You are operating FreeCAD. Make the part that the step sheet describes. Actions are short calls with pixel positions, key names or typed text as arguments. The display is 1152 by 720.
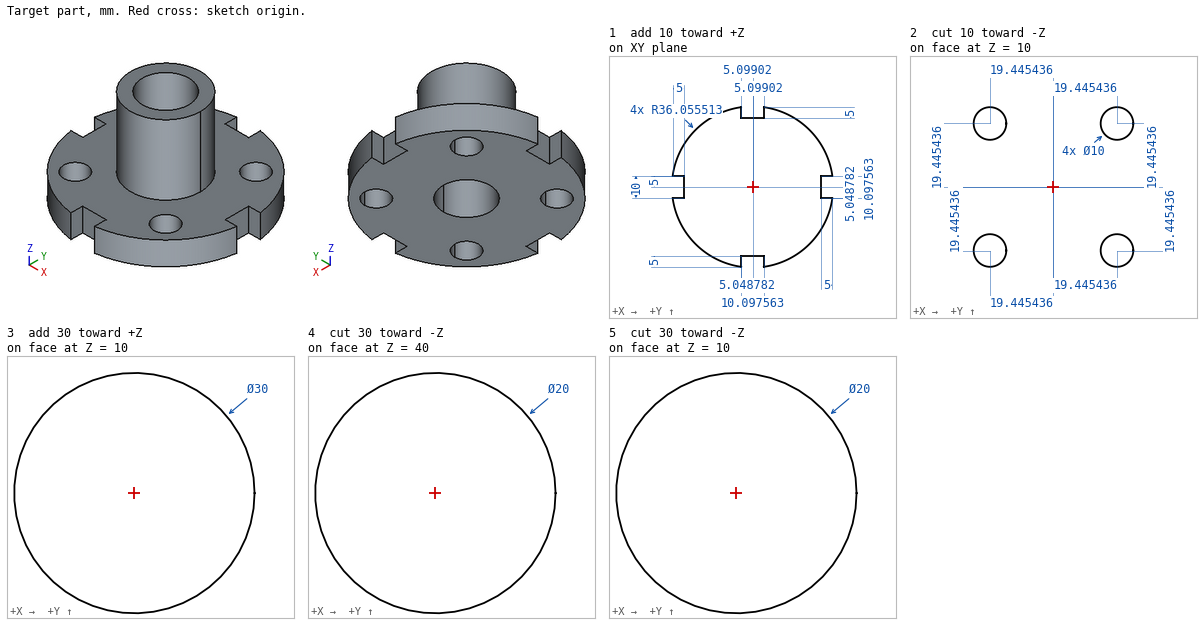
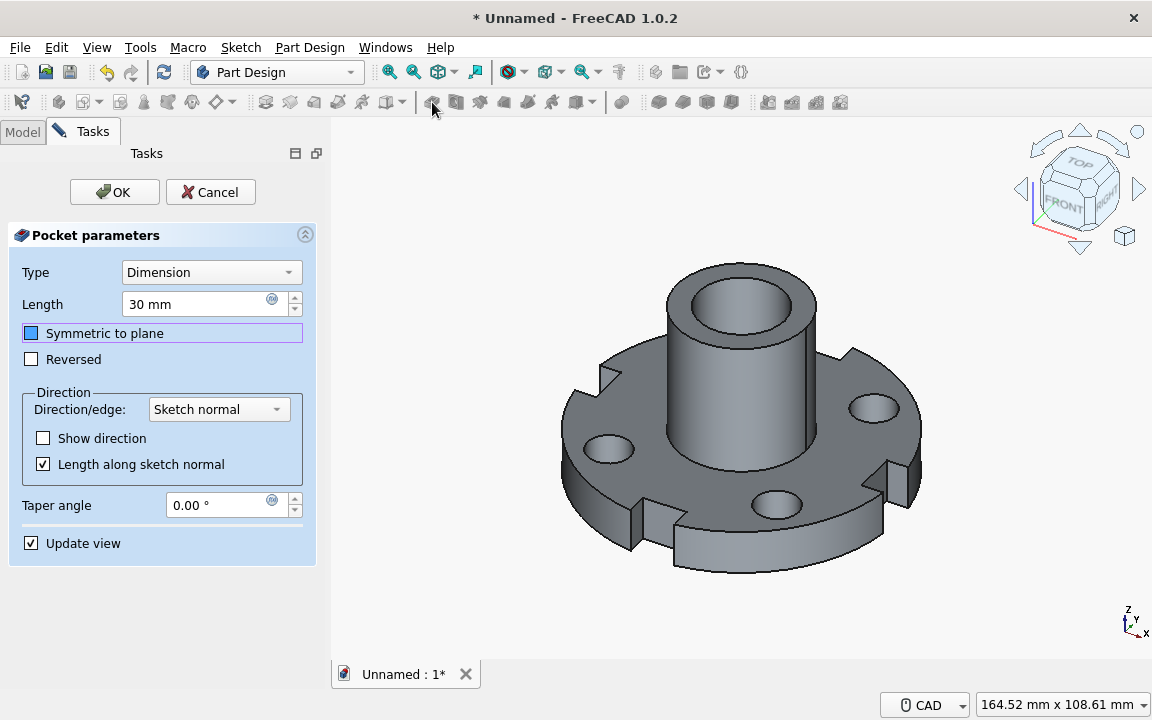
click(115, 192)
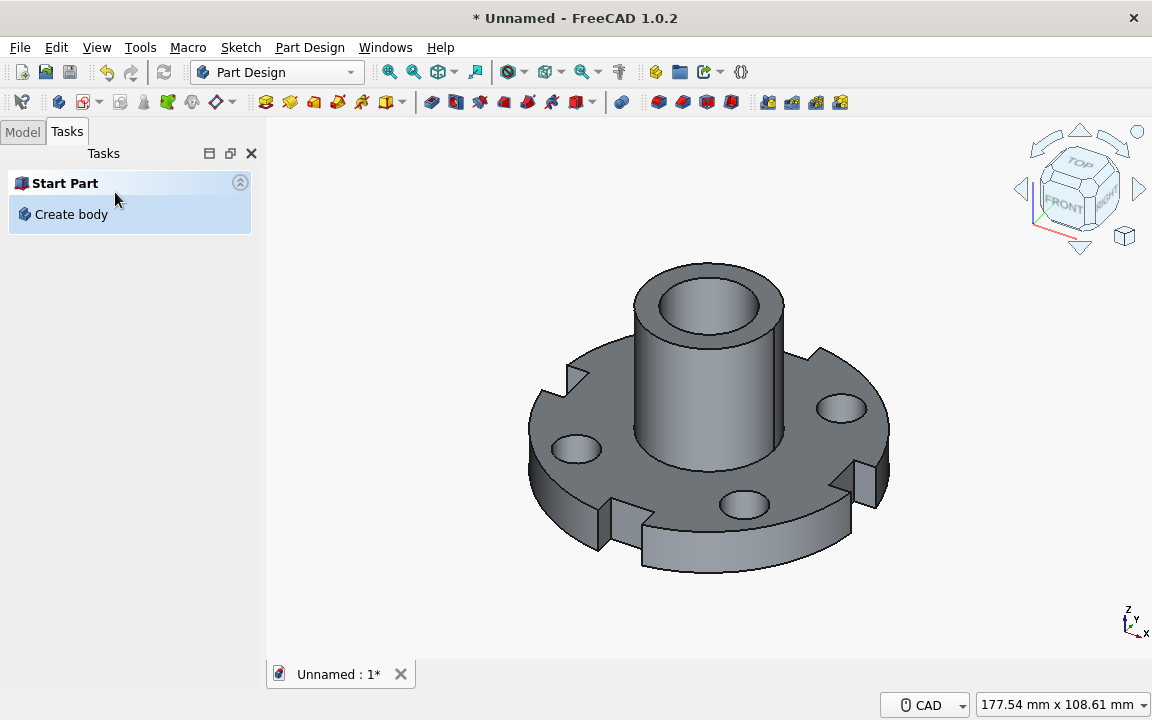
click(621, 399)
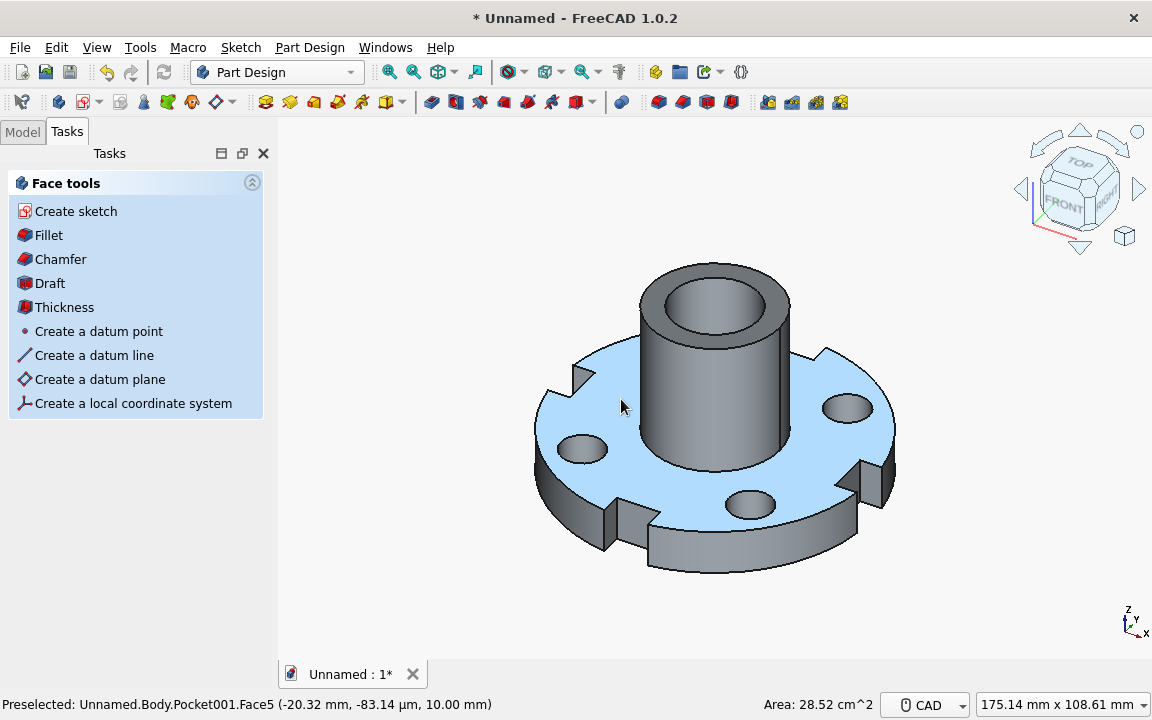
click(84, 102)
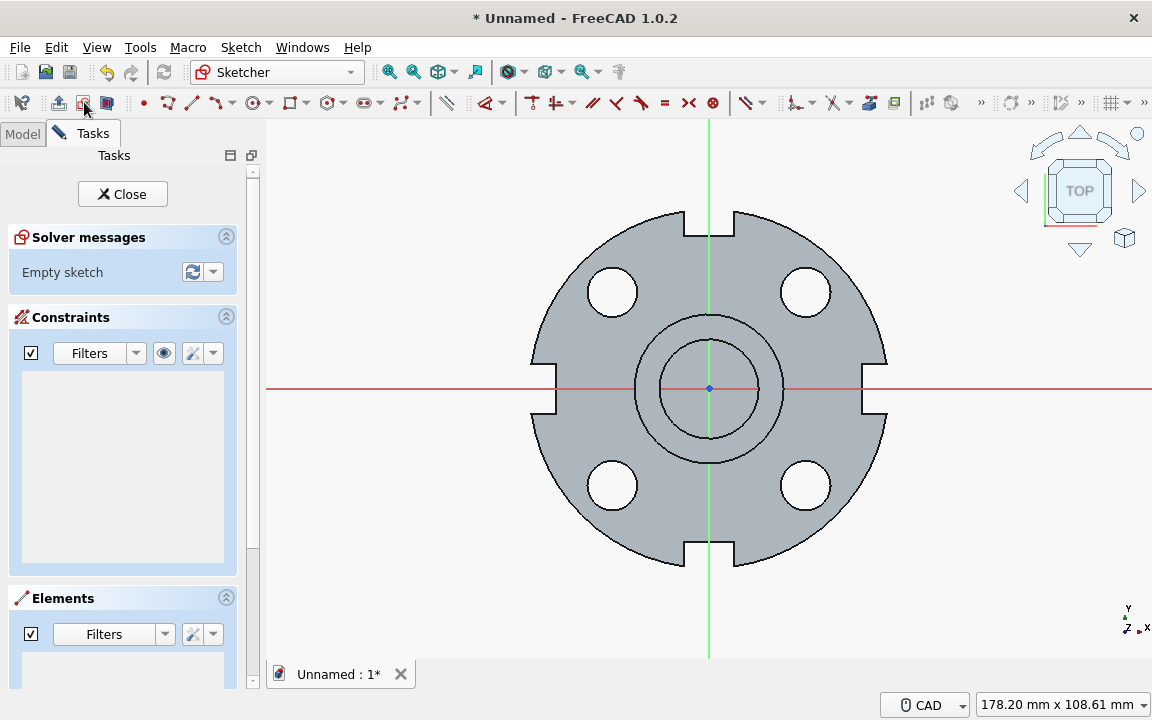
scroll(739, 389, up, 6)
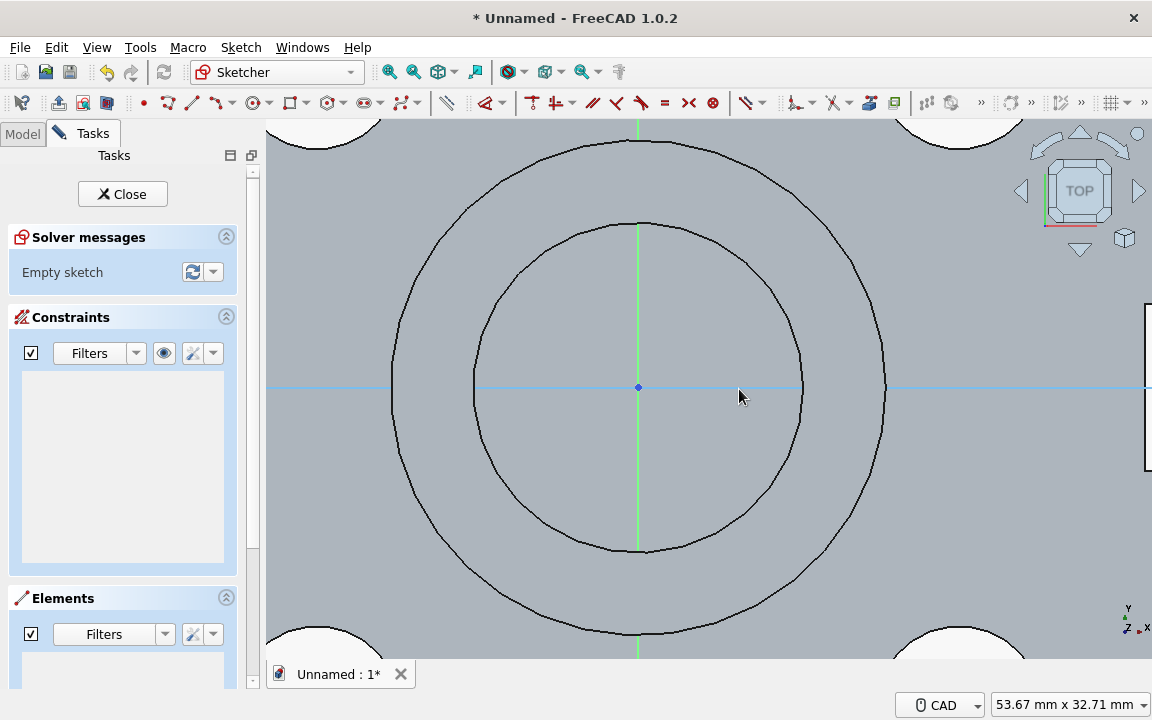
click(254, 104)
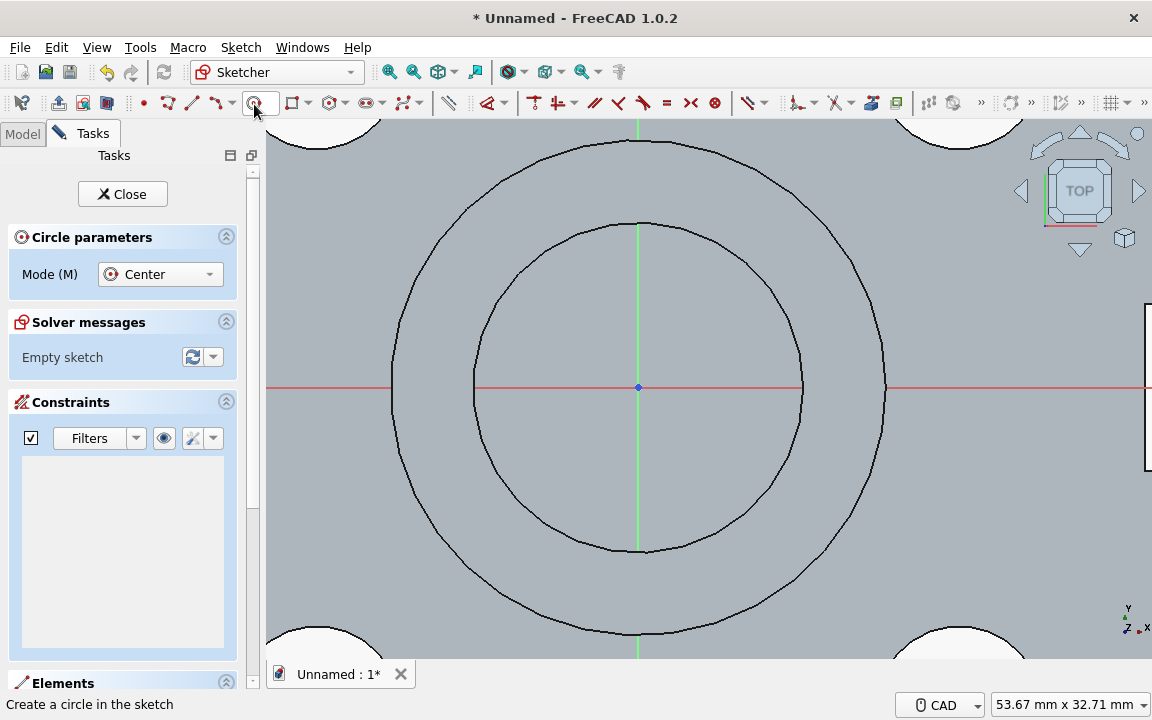
click(638, 388)
move(755, 271)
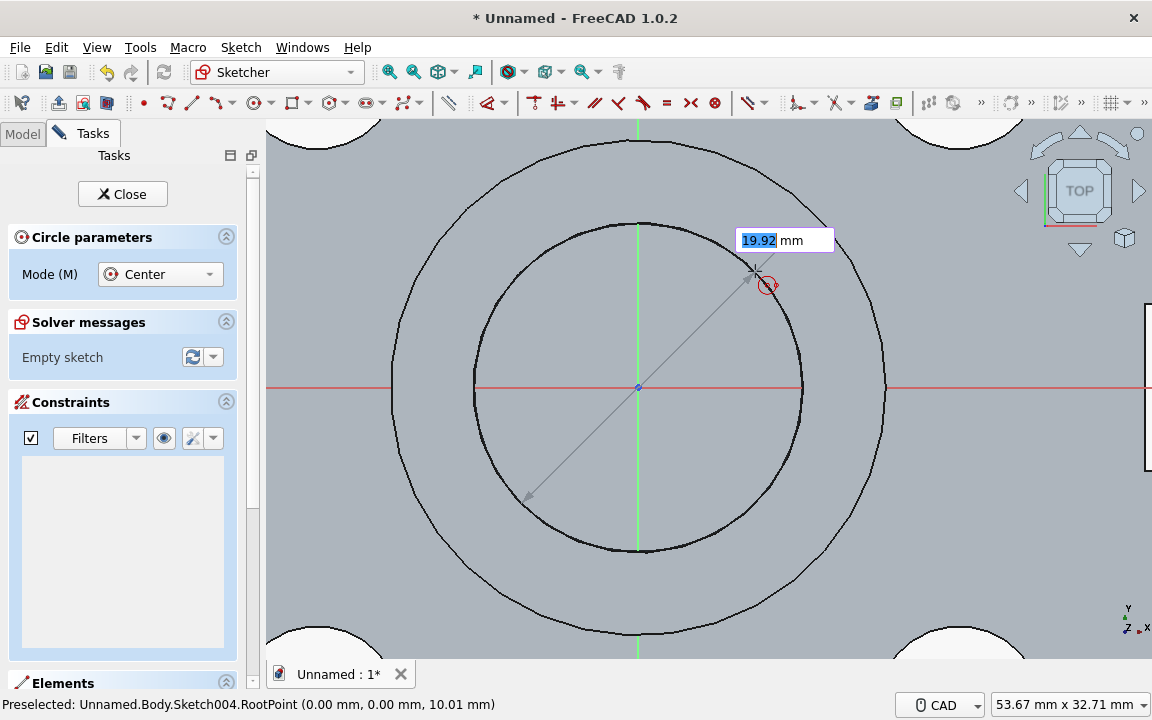
text(20)
key(Return)
key(Escape)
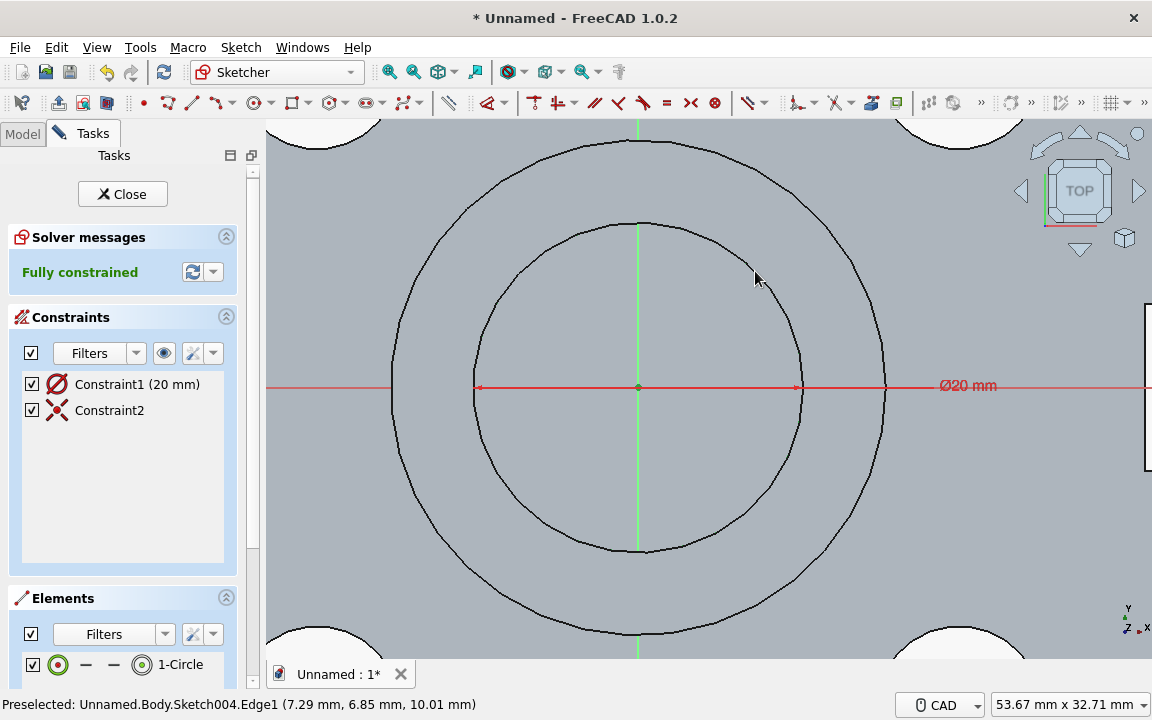
click(123, 194)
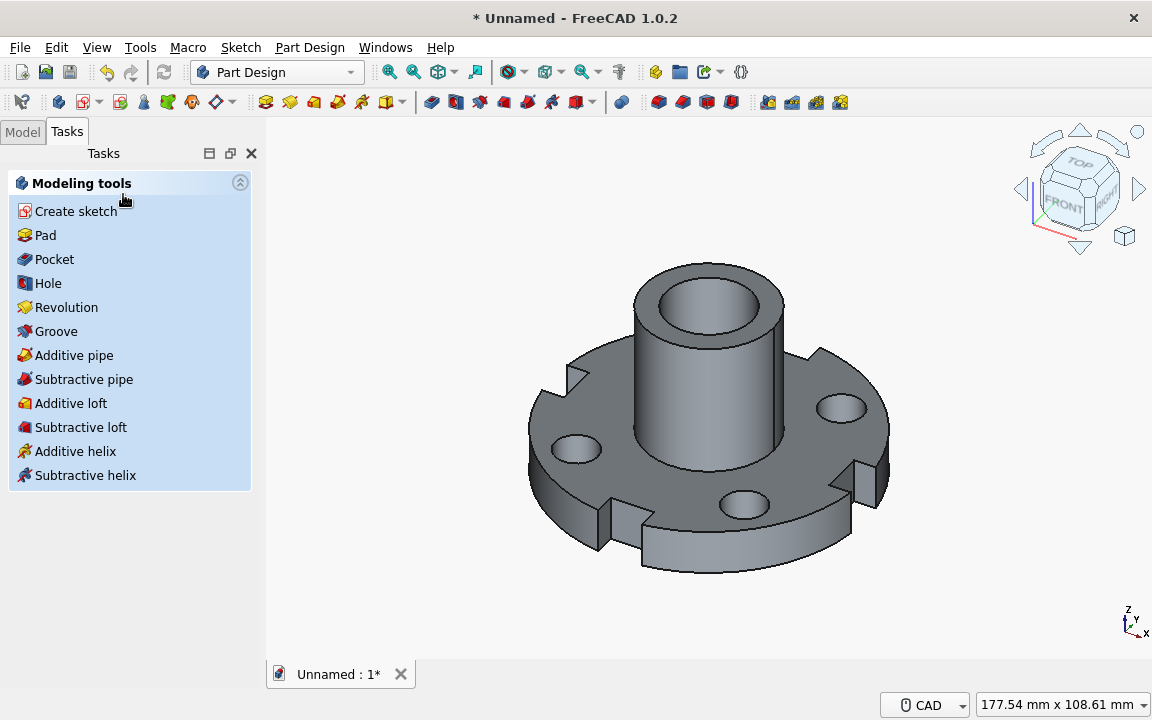
click(432, 102)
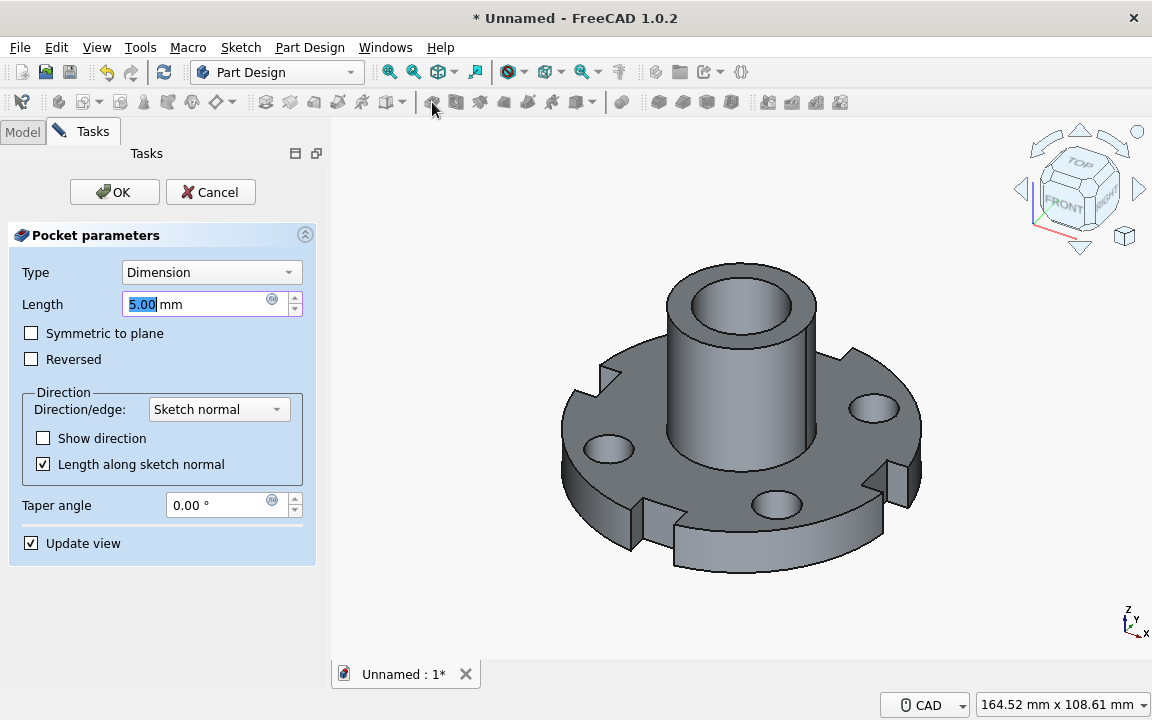
text(30)
key(Tab)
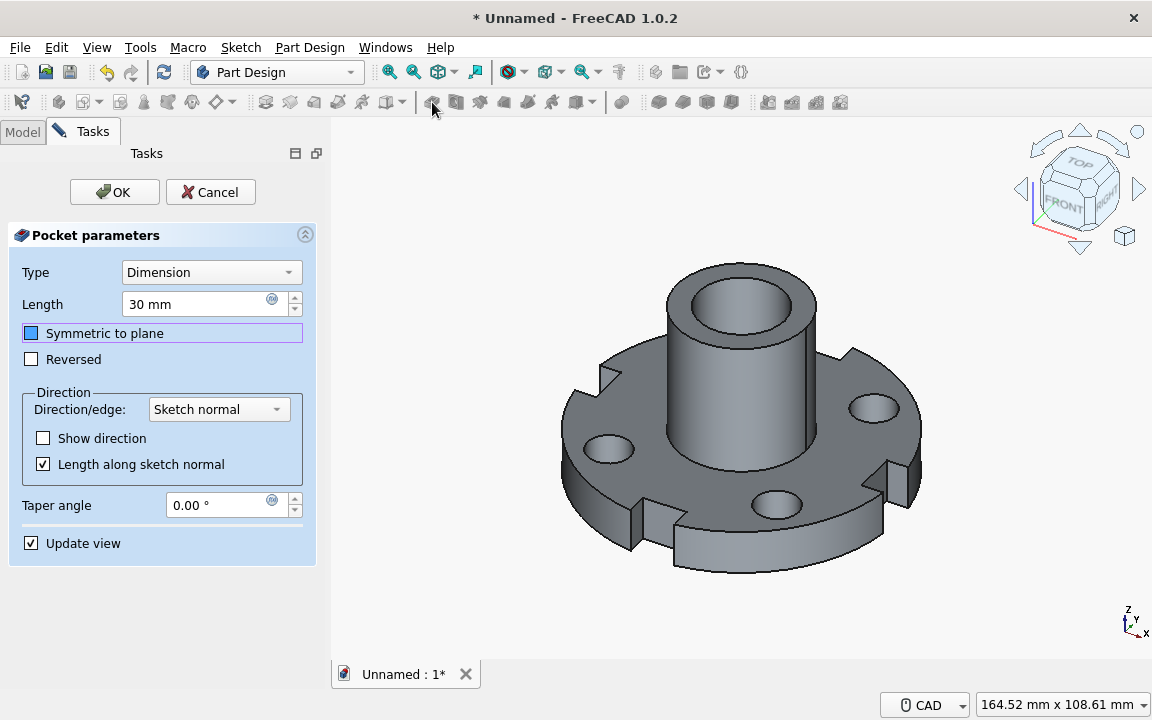
click(115, 192)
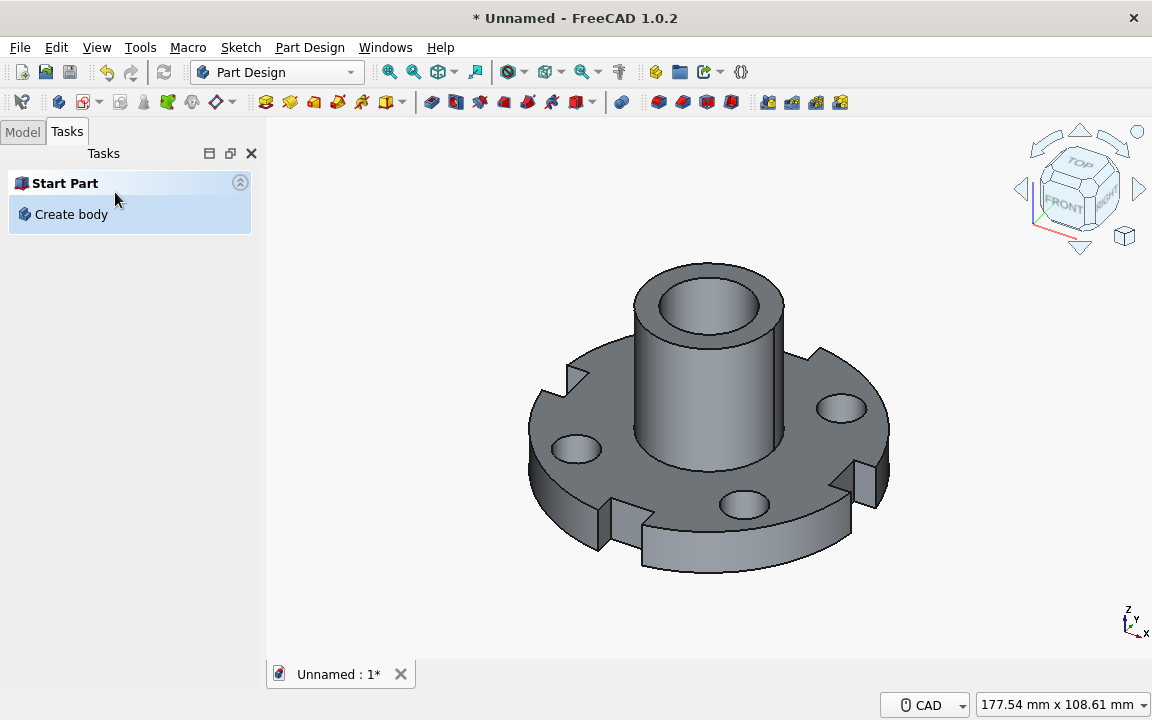
key(0)